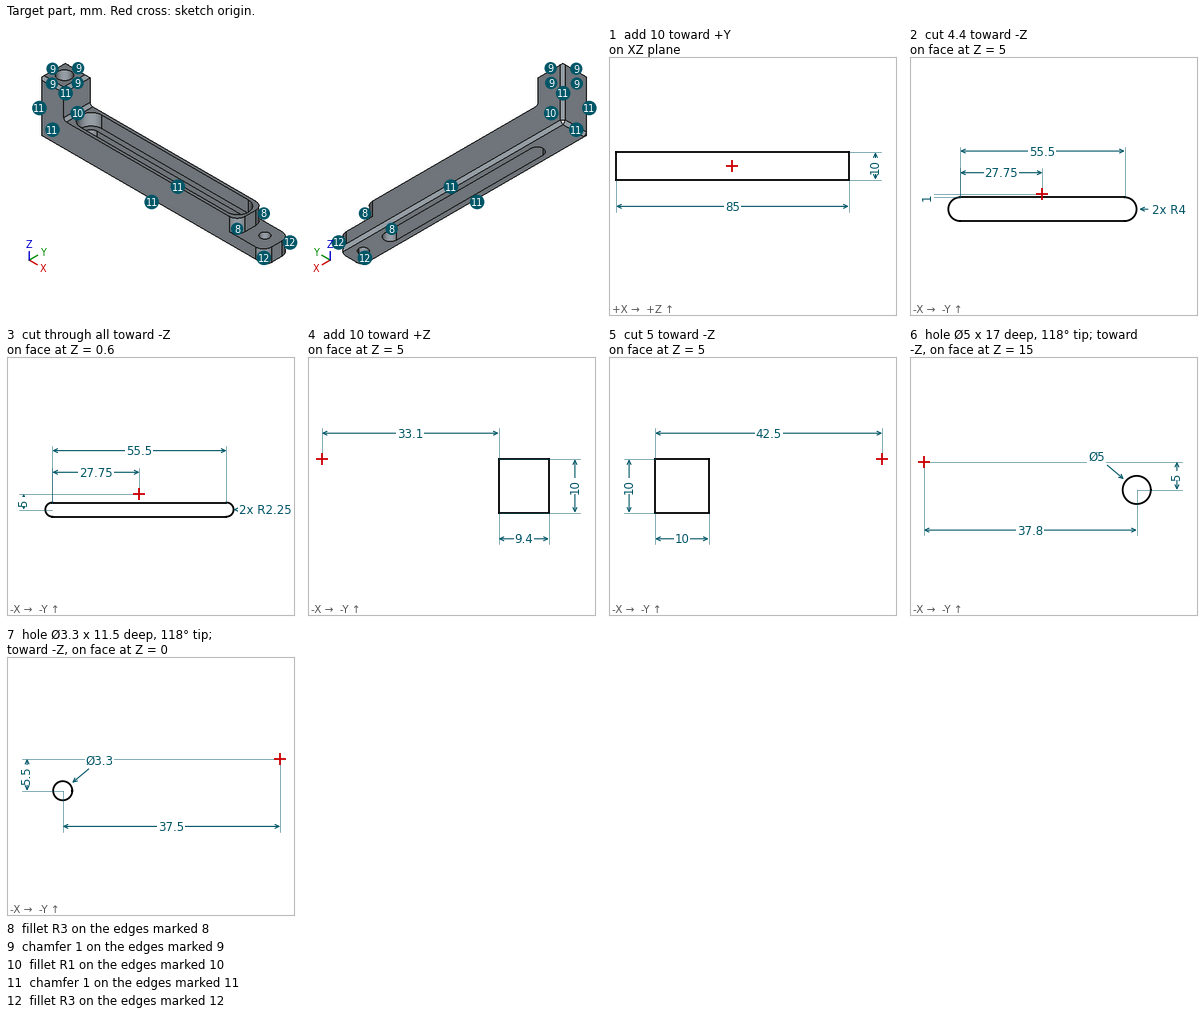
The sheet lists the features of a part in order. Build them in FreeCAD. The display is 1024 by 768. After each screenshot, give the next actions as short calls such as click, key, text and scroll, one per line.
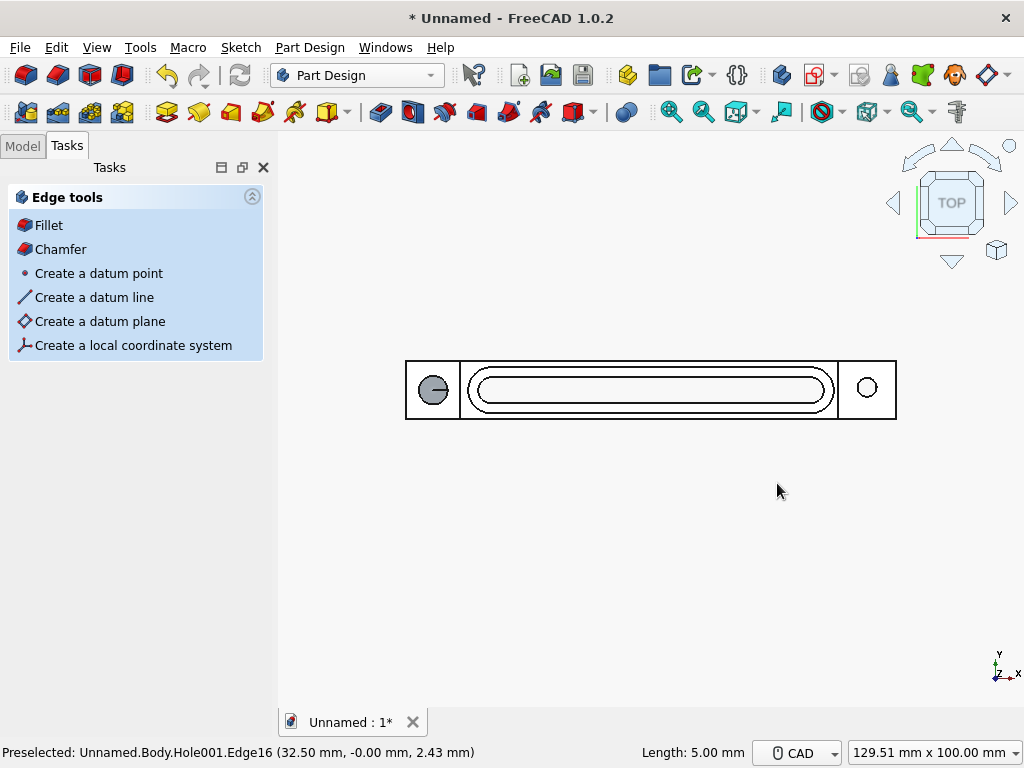
key(1)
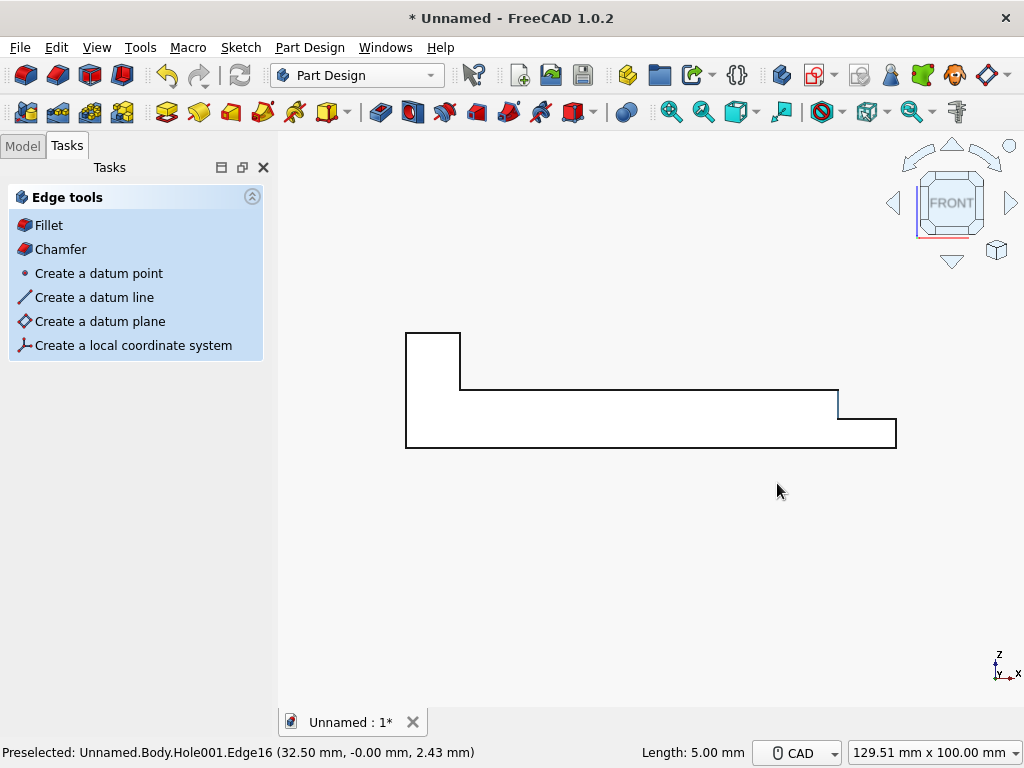
key(3)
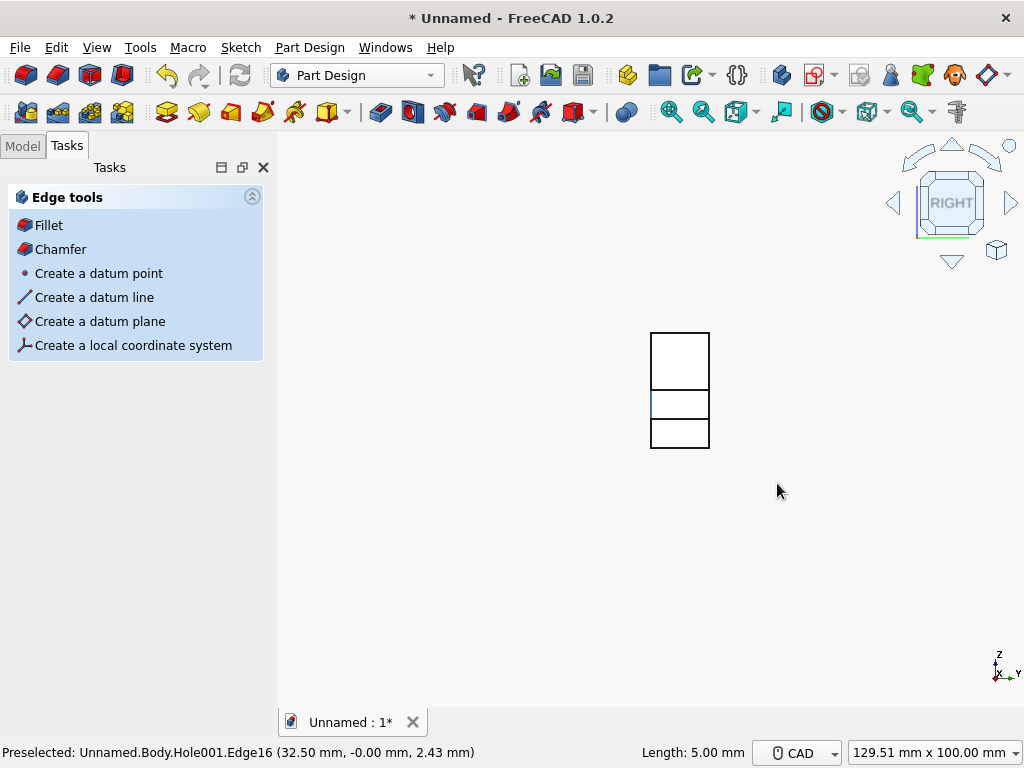
key(v)
key(f)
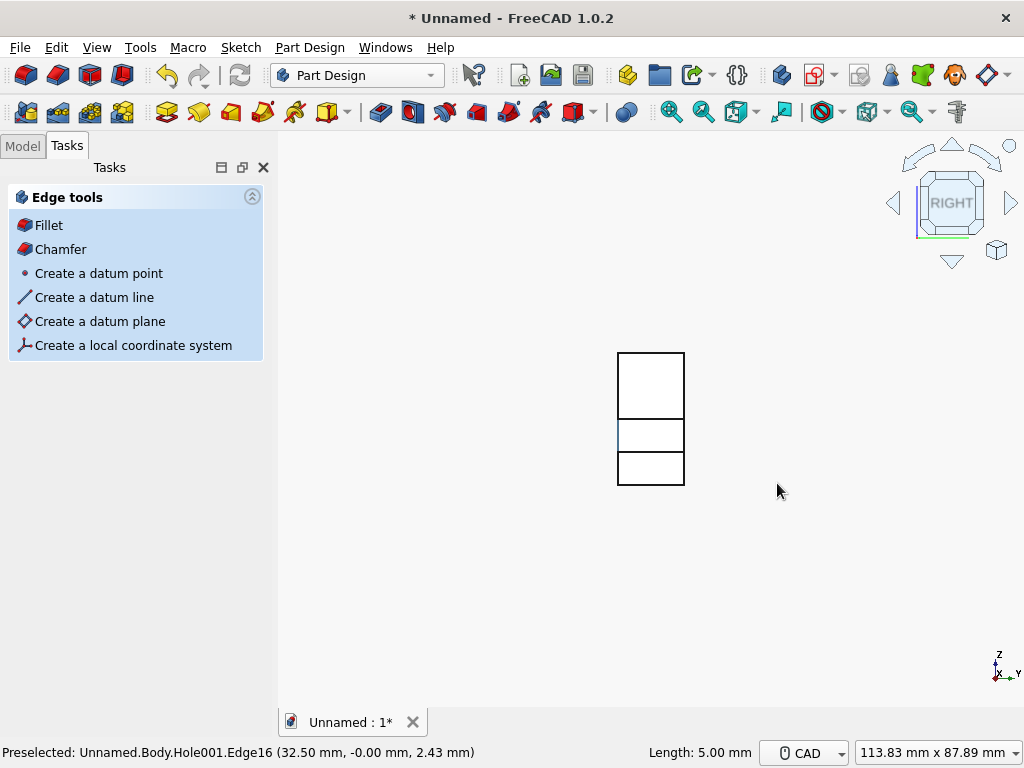
click(684, 434, ctrl)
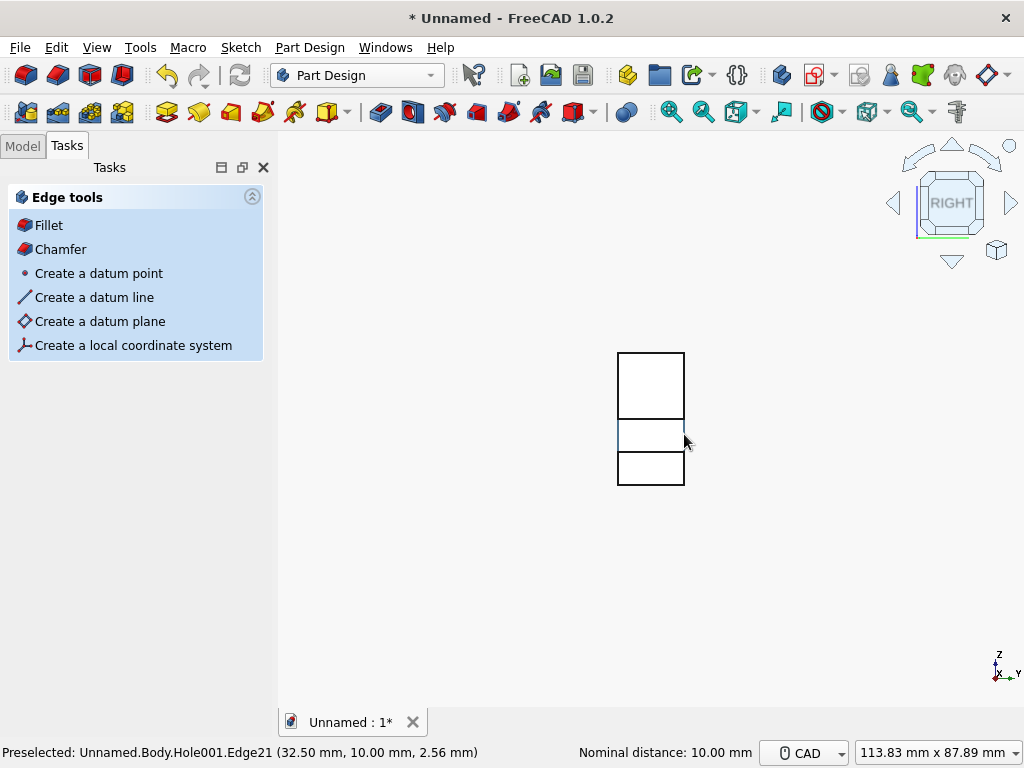
click(26, 76)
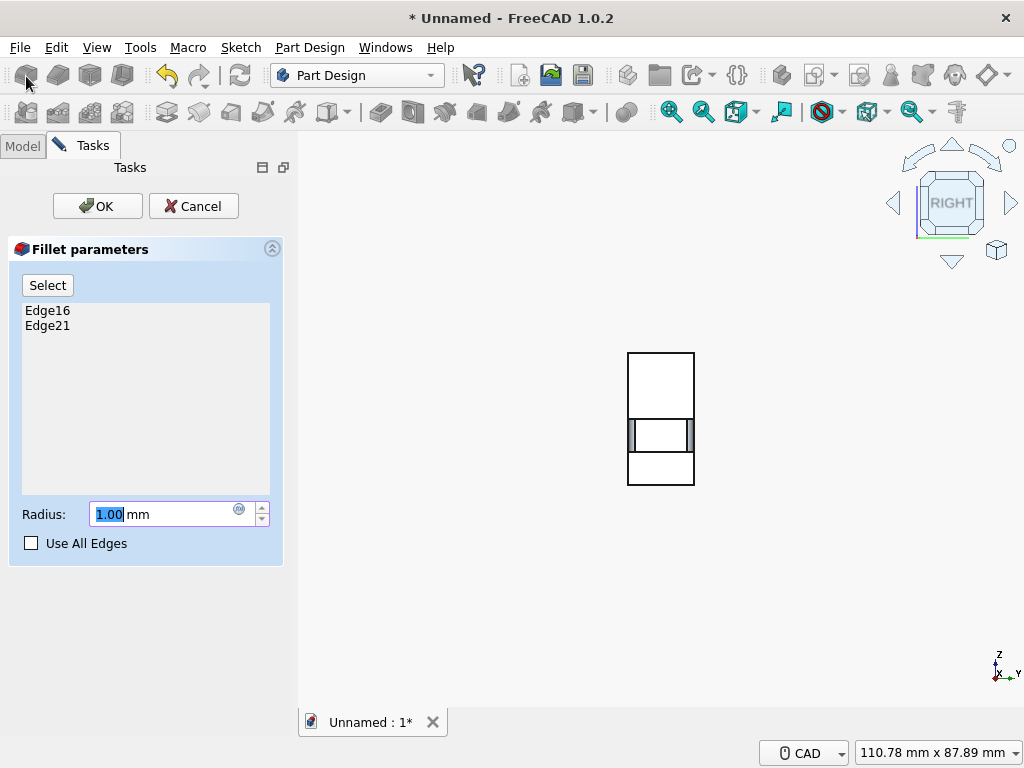
text(3)
key(Tab)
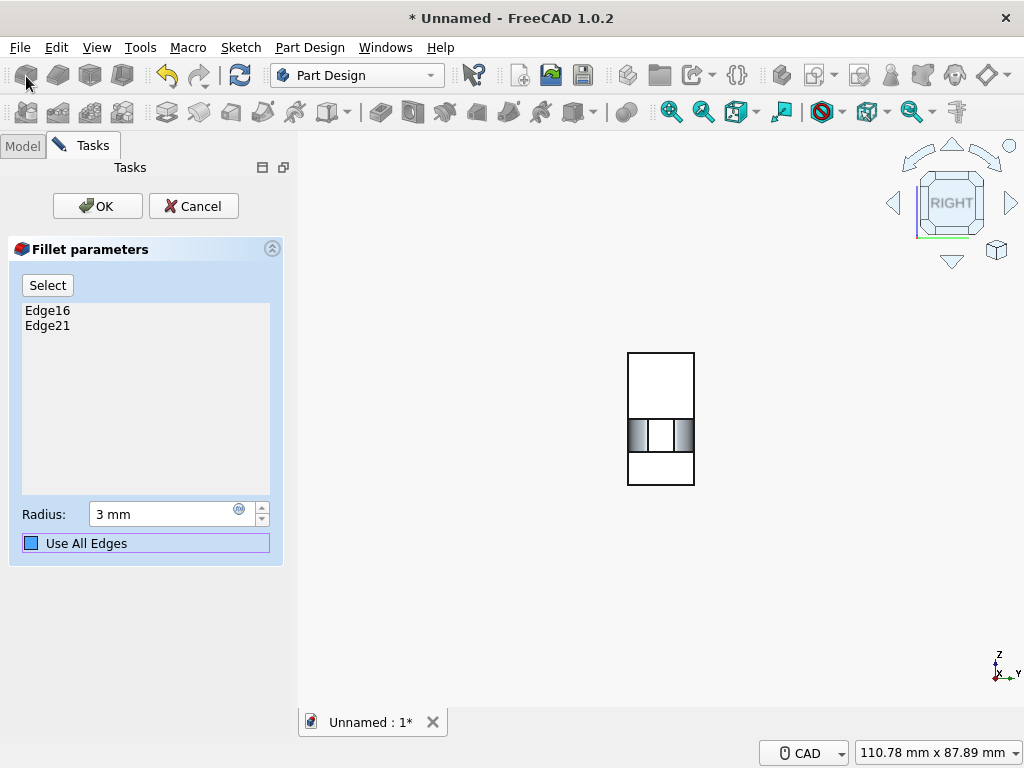
click(98, 206)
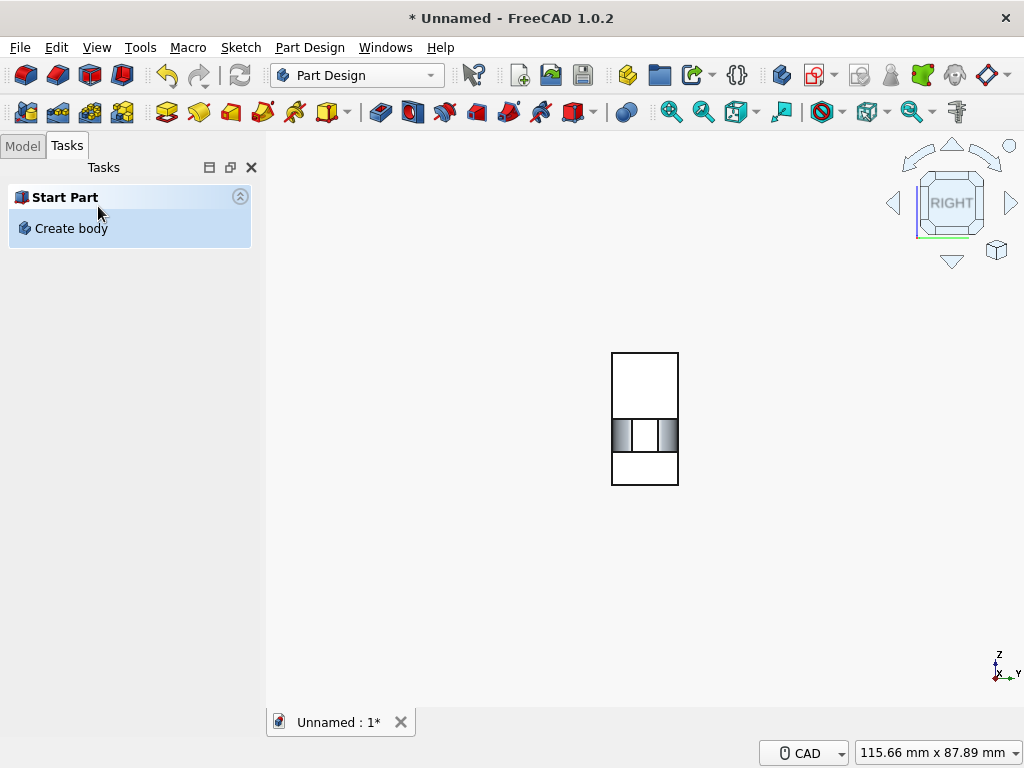
click(672, 112)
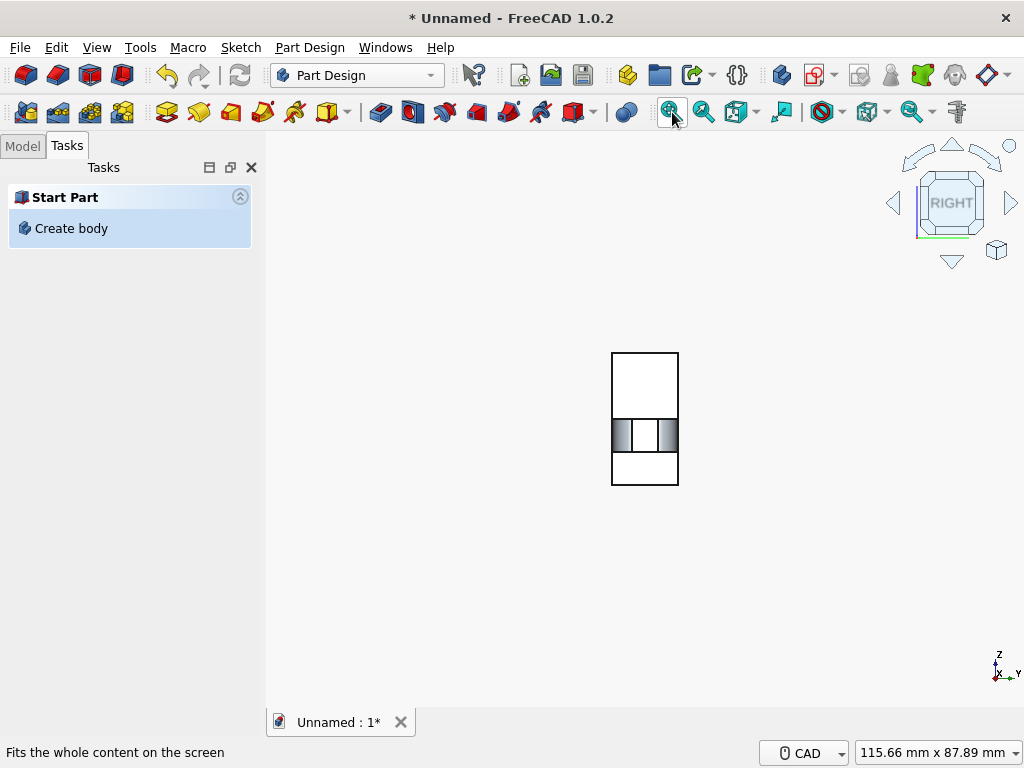
click(645, 352)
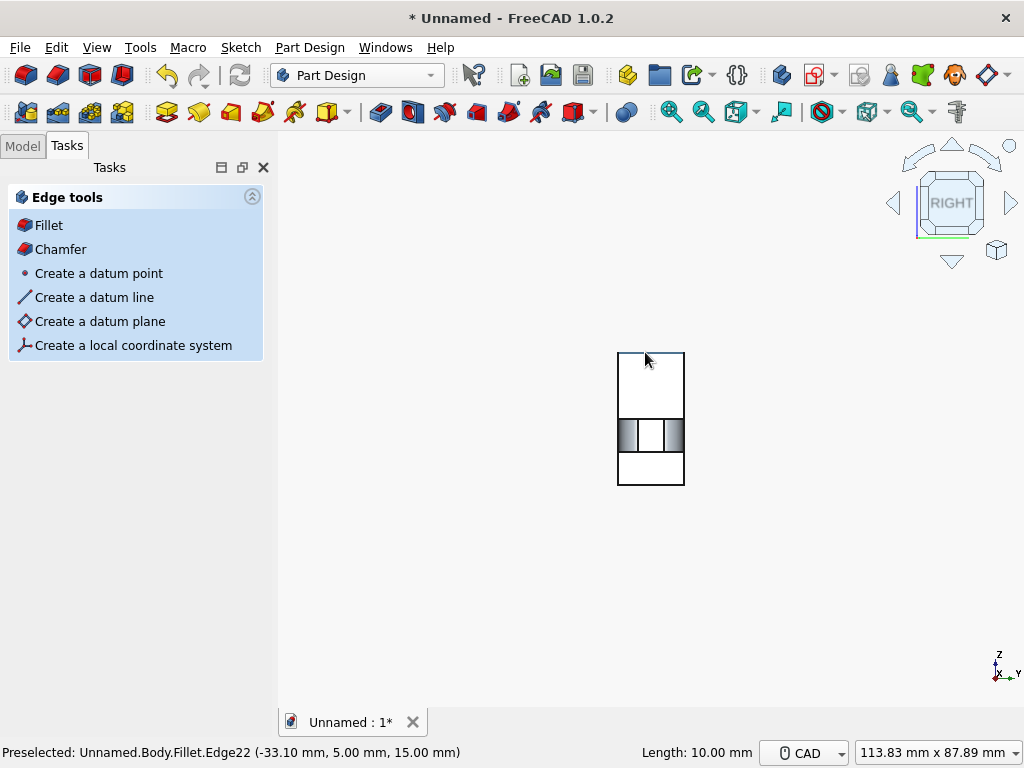
key(0)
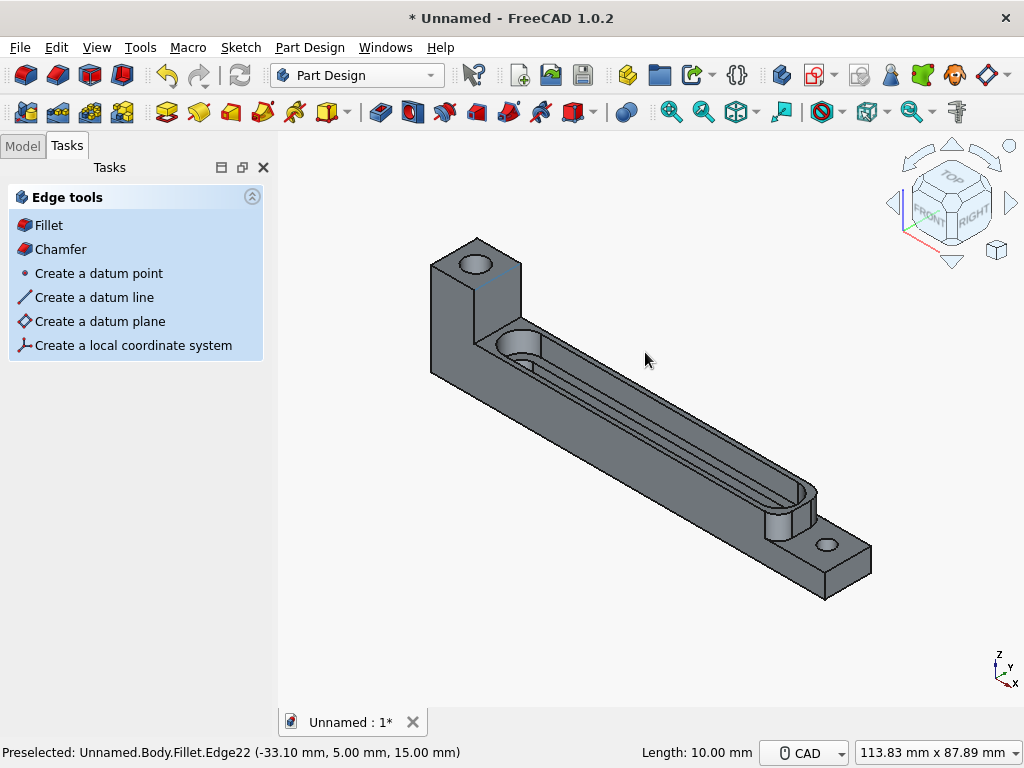
click(453, 277, ctrl)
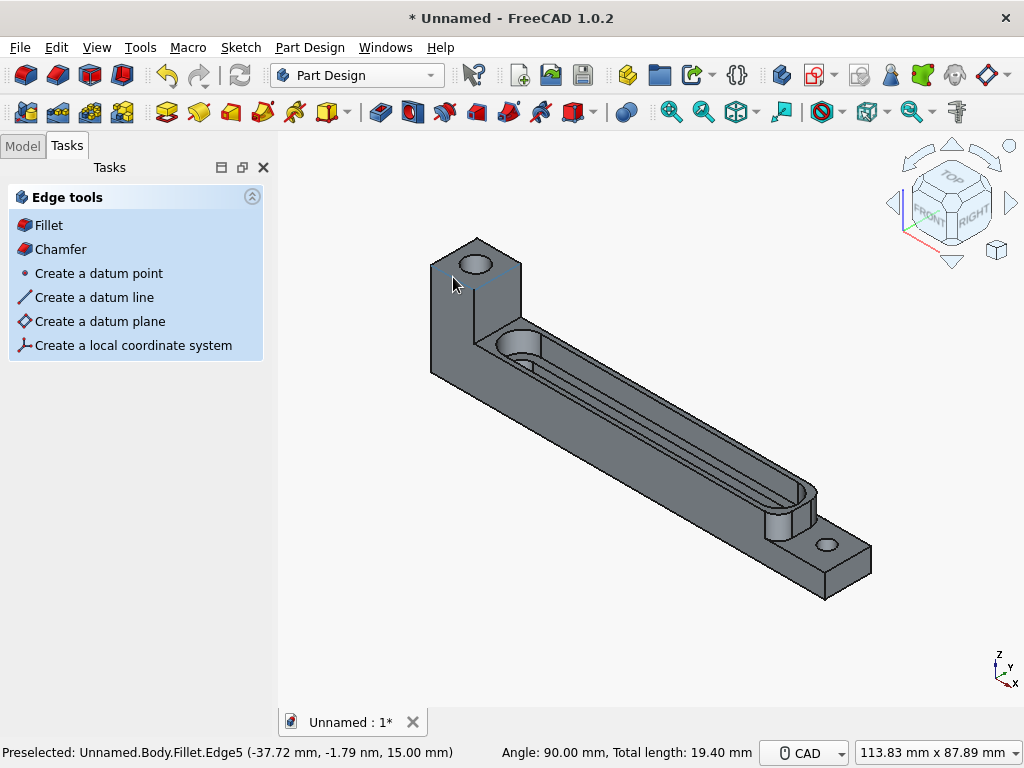
key(2)